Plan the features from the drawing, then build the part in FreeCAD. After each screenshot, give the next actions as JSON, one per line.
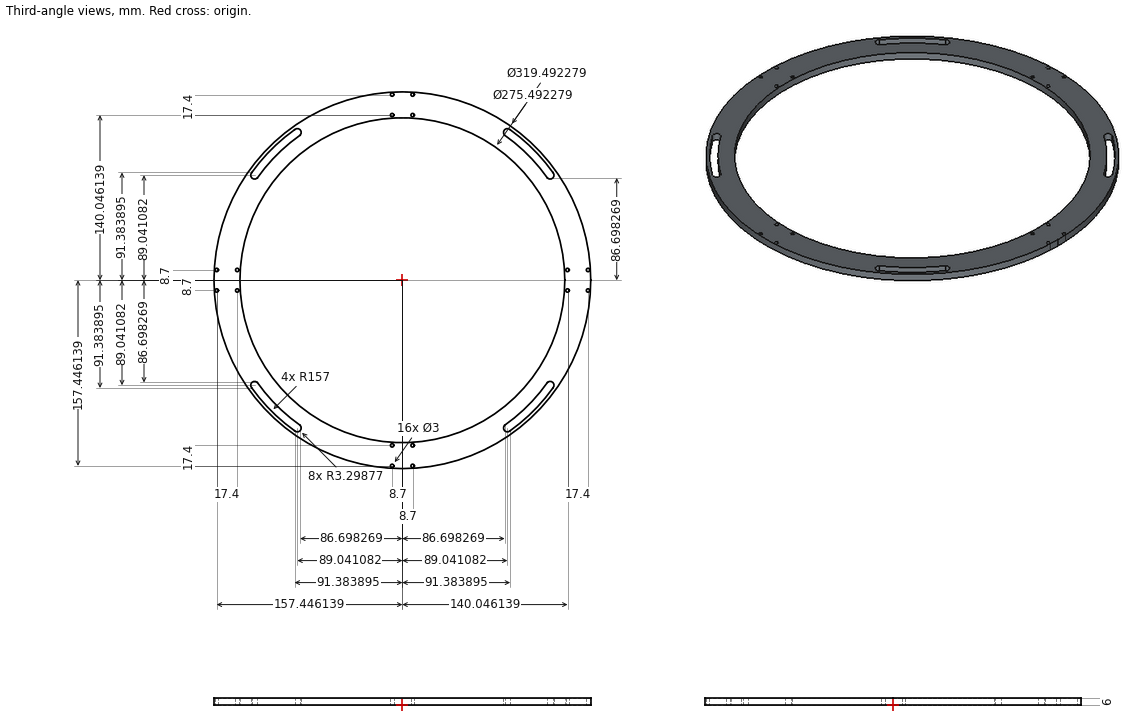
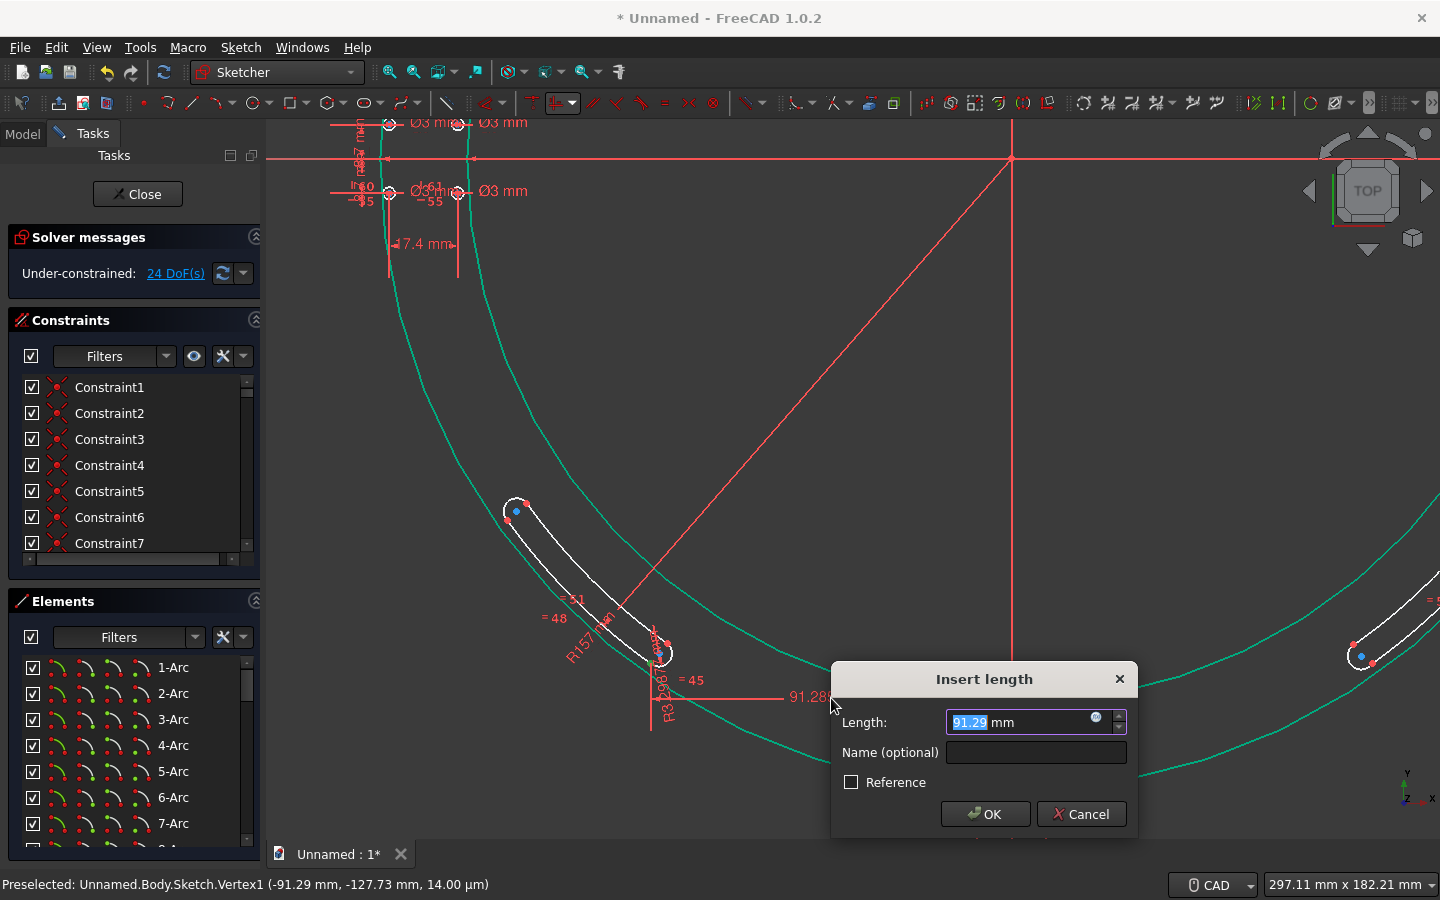
{"action": "type", "text": "91.383895"}
{"action": "key", "text": "Return"}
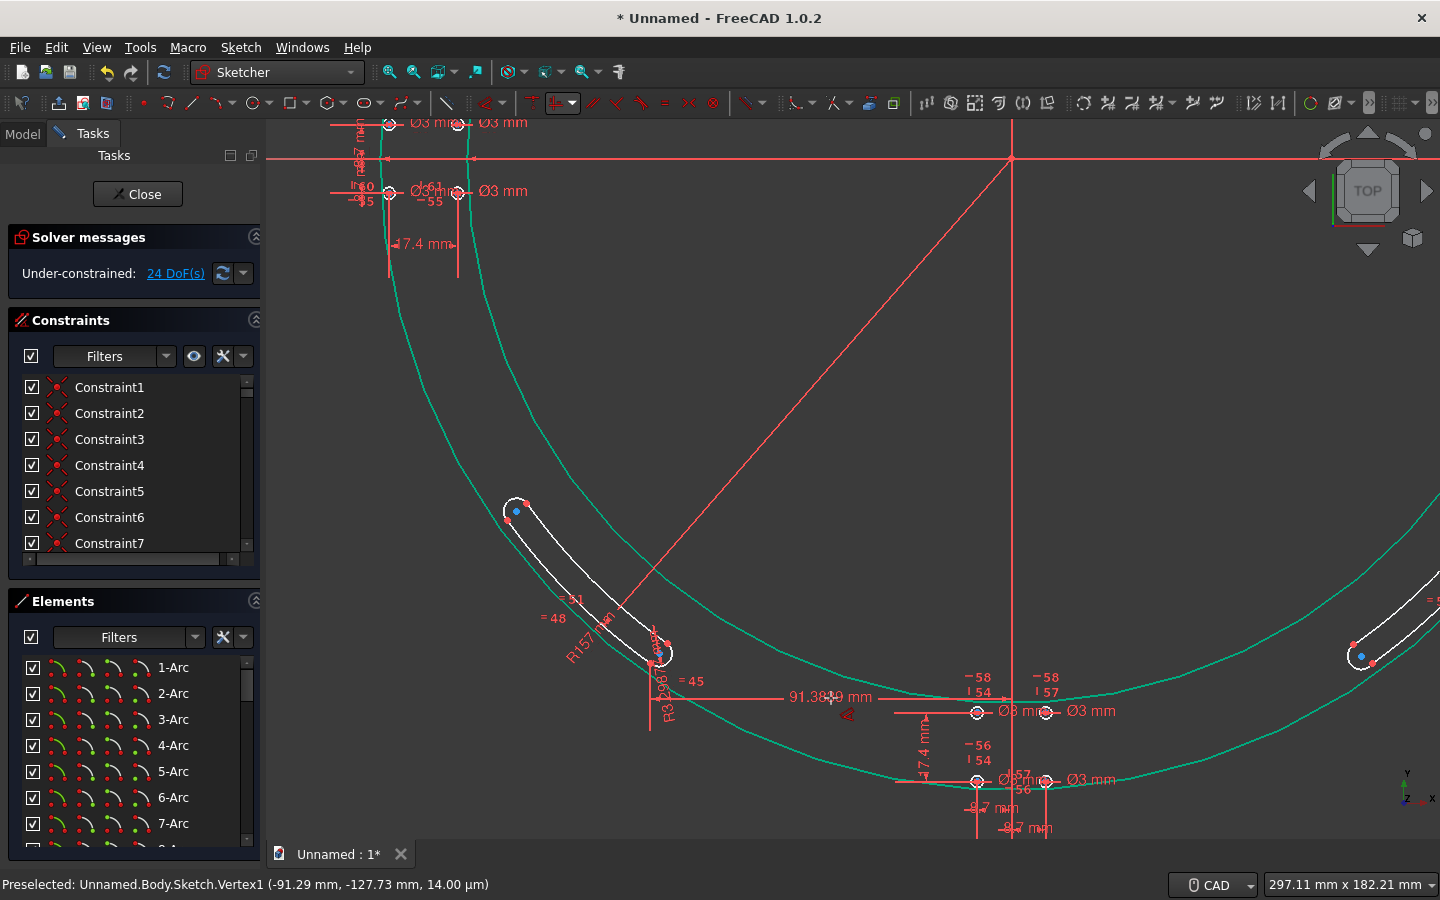
{"action": "left_click", "coordinate": [668, 644]}
{"action": "left_click", "coordinate": [761, 678]}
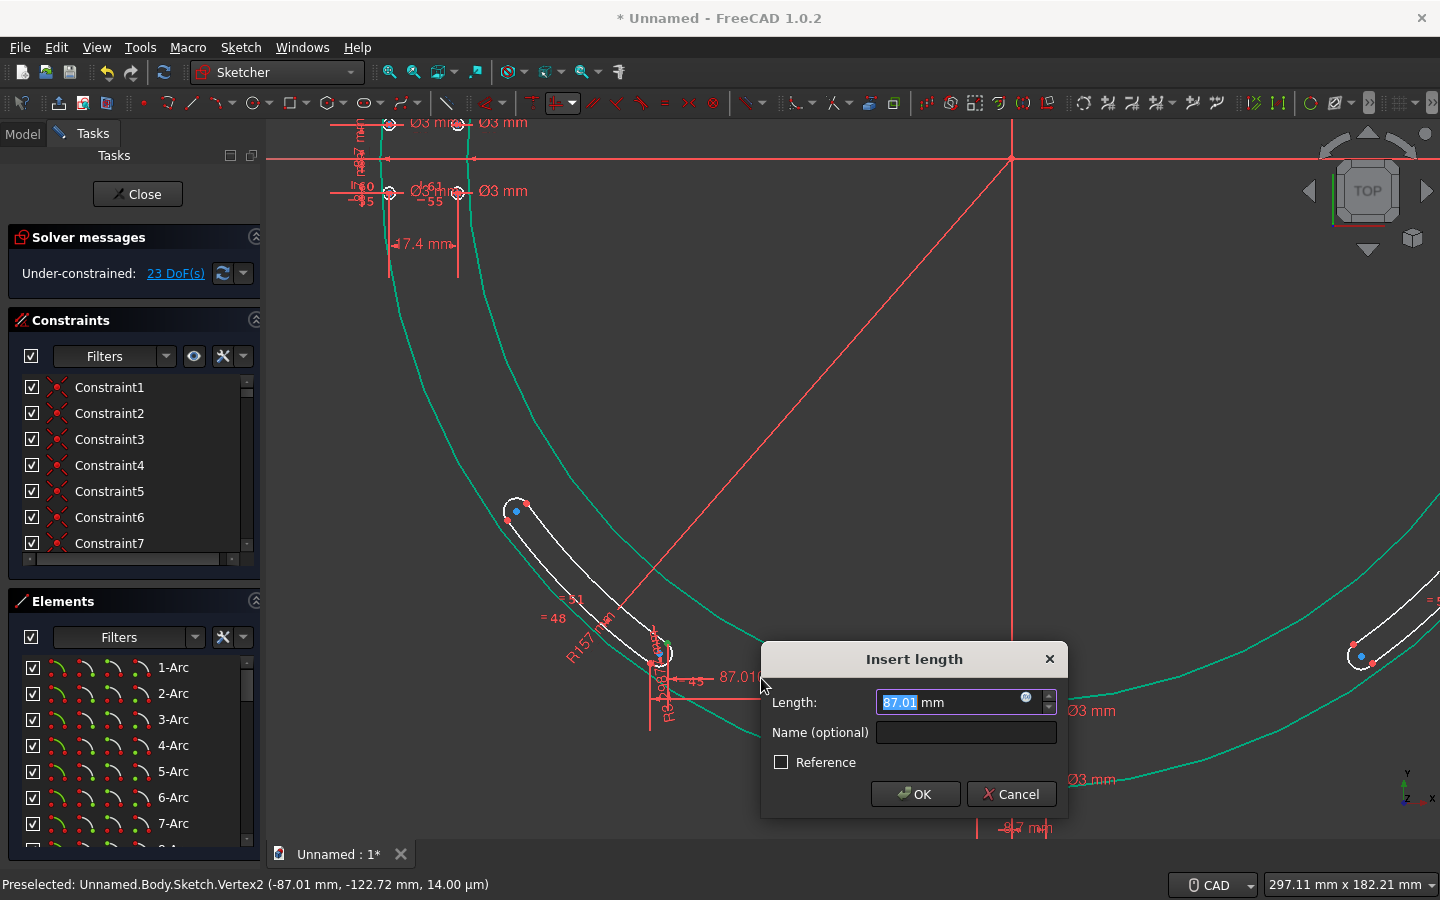
{"action": "type", "text": "86.698269"}
{"action": "key", "text": "Return"}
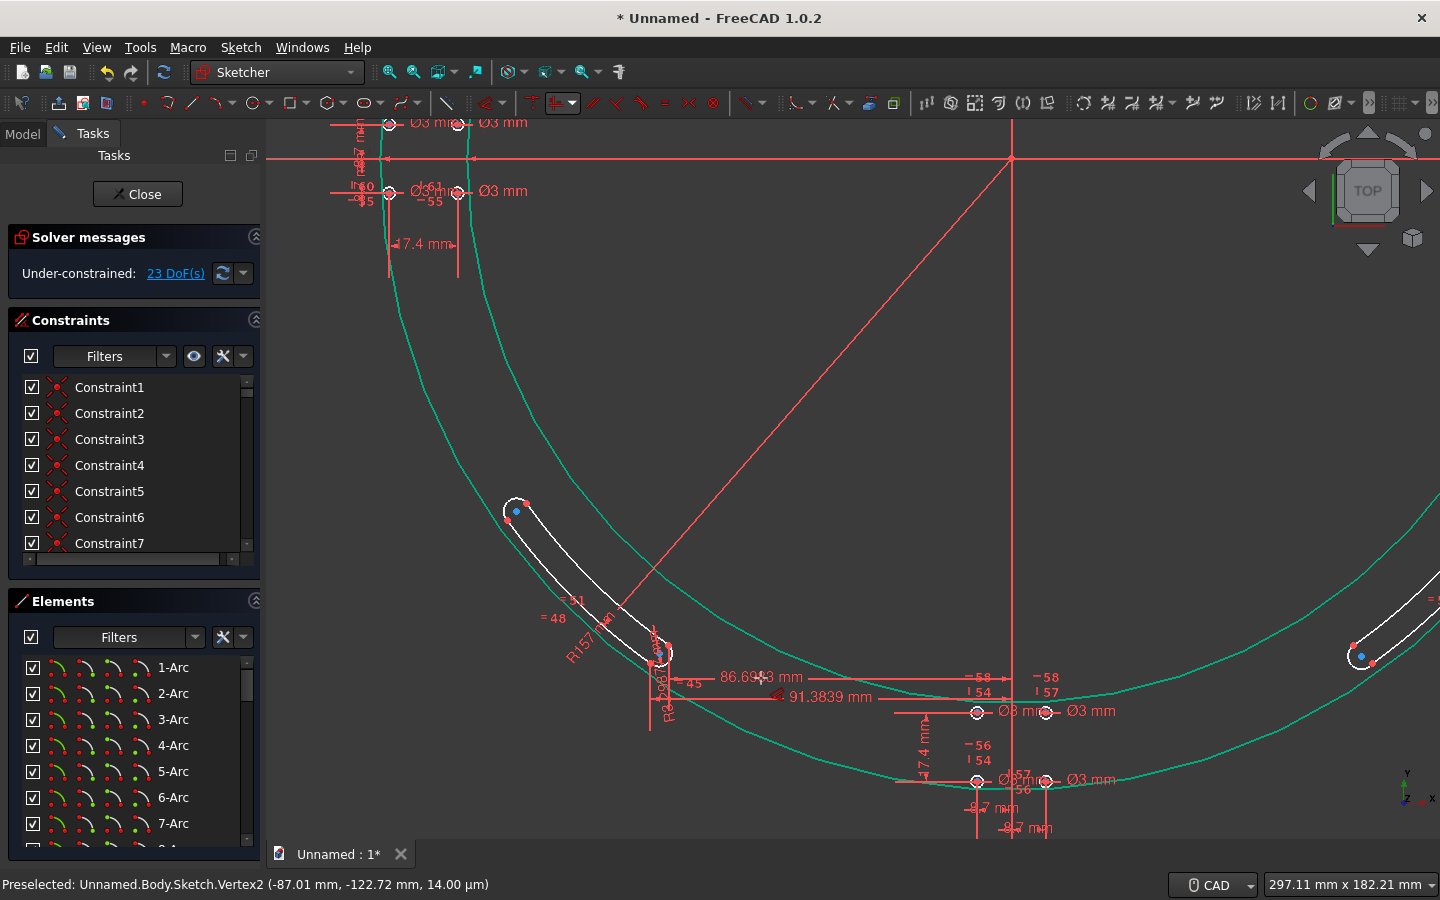
{"action": "left_click", "coordinate": [508, 521]}
{"action": "left_click", "coordinate": [474, 340]}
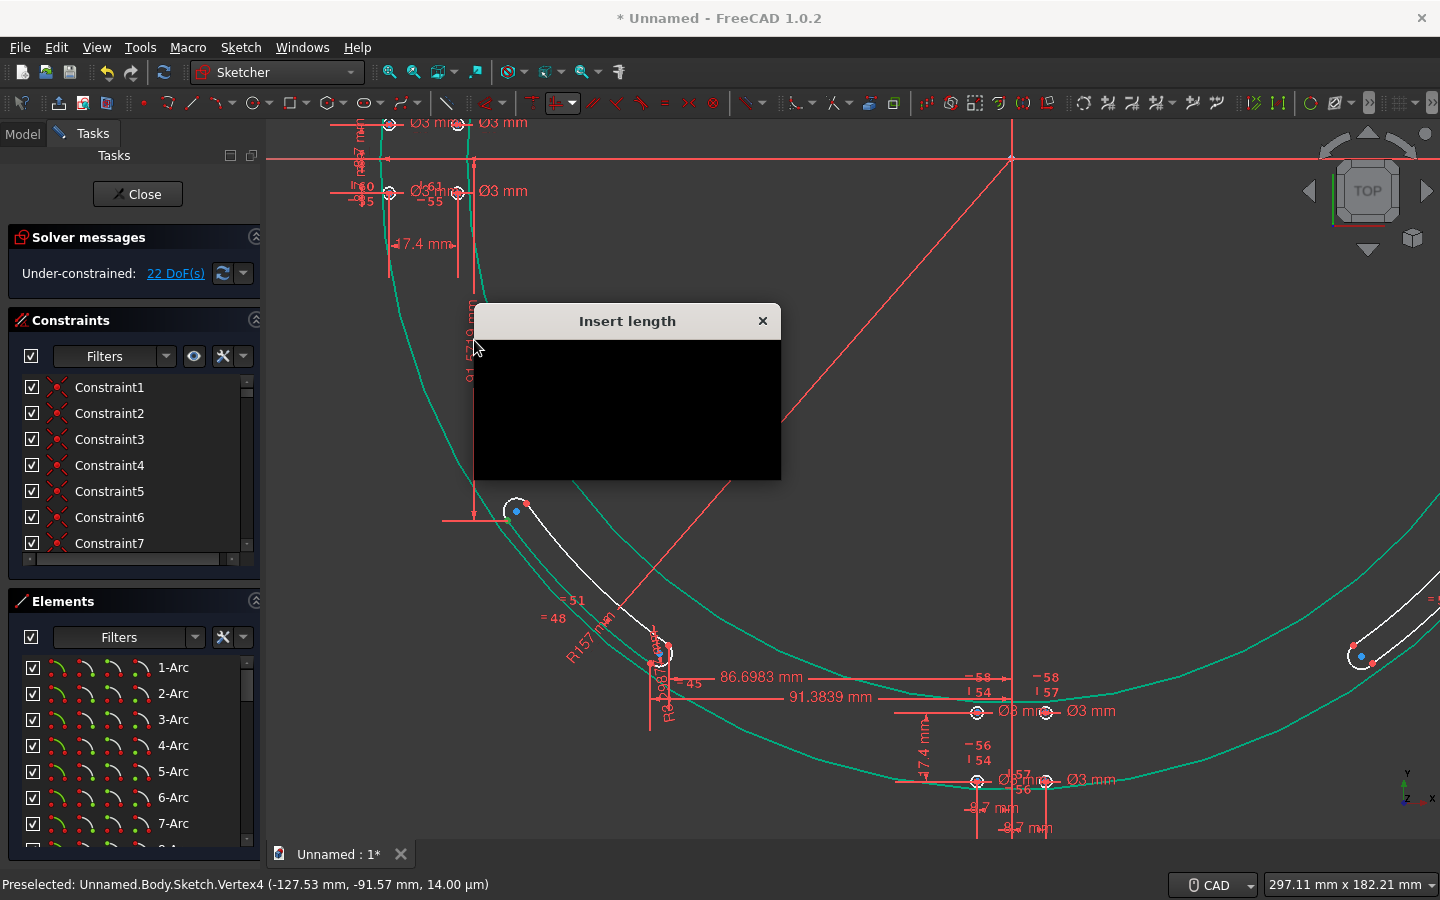
{"action": "type", "text": "91.383895"}
{"action": "key", "text": "Return"}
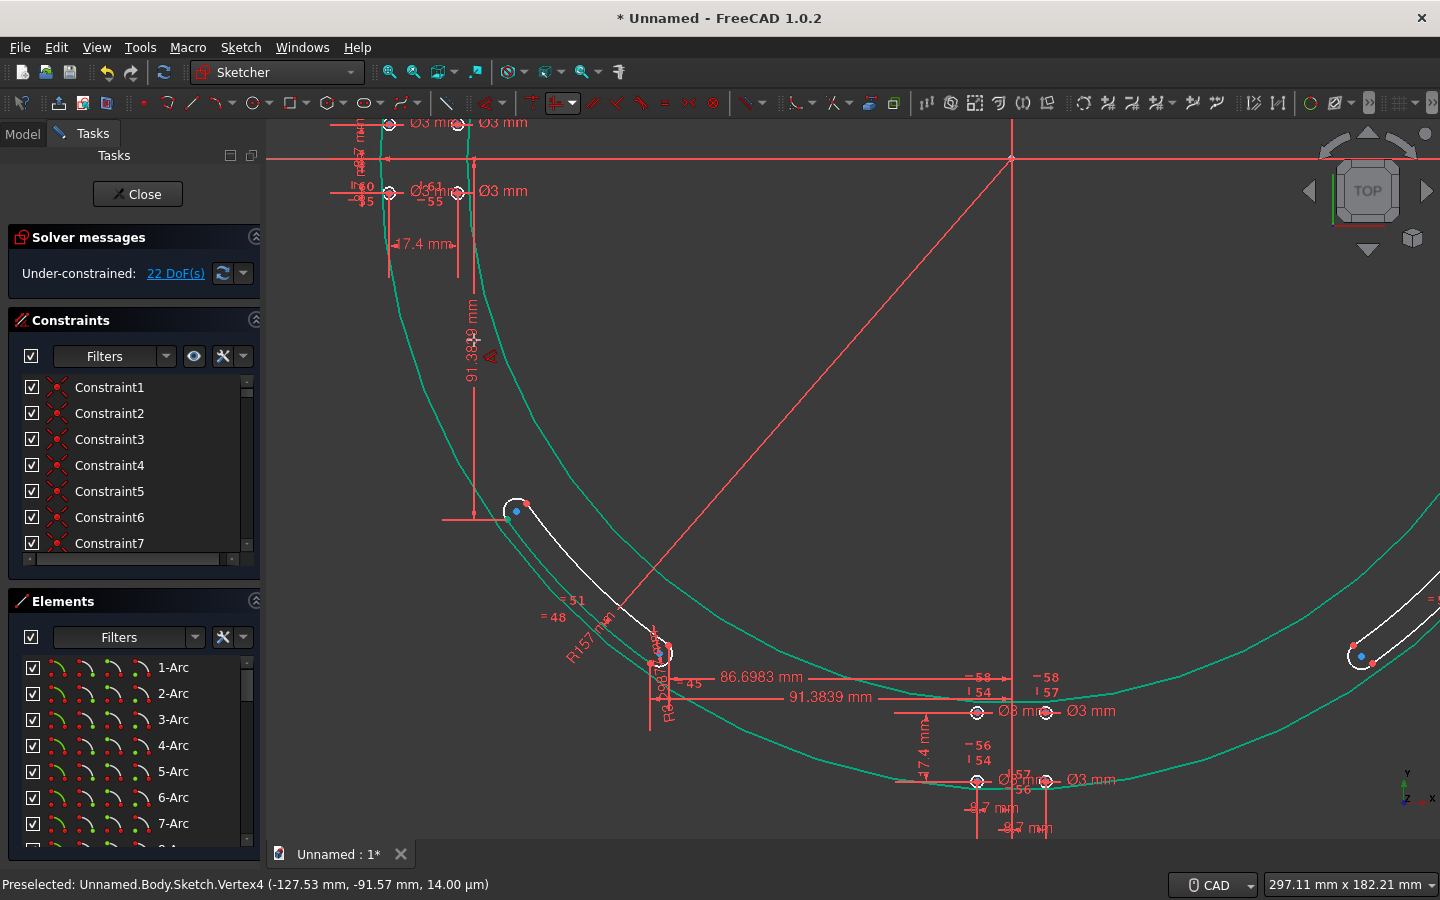
{"action": "left_click", "coordinate": [526, 503]}
{"action": "left_click", "coordinate": [492, 410]}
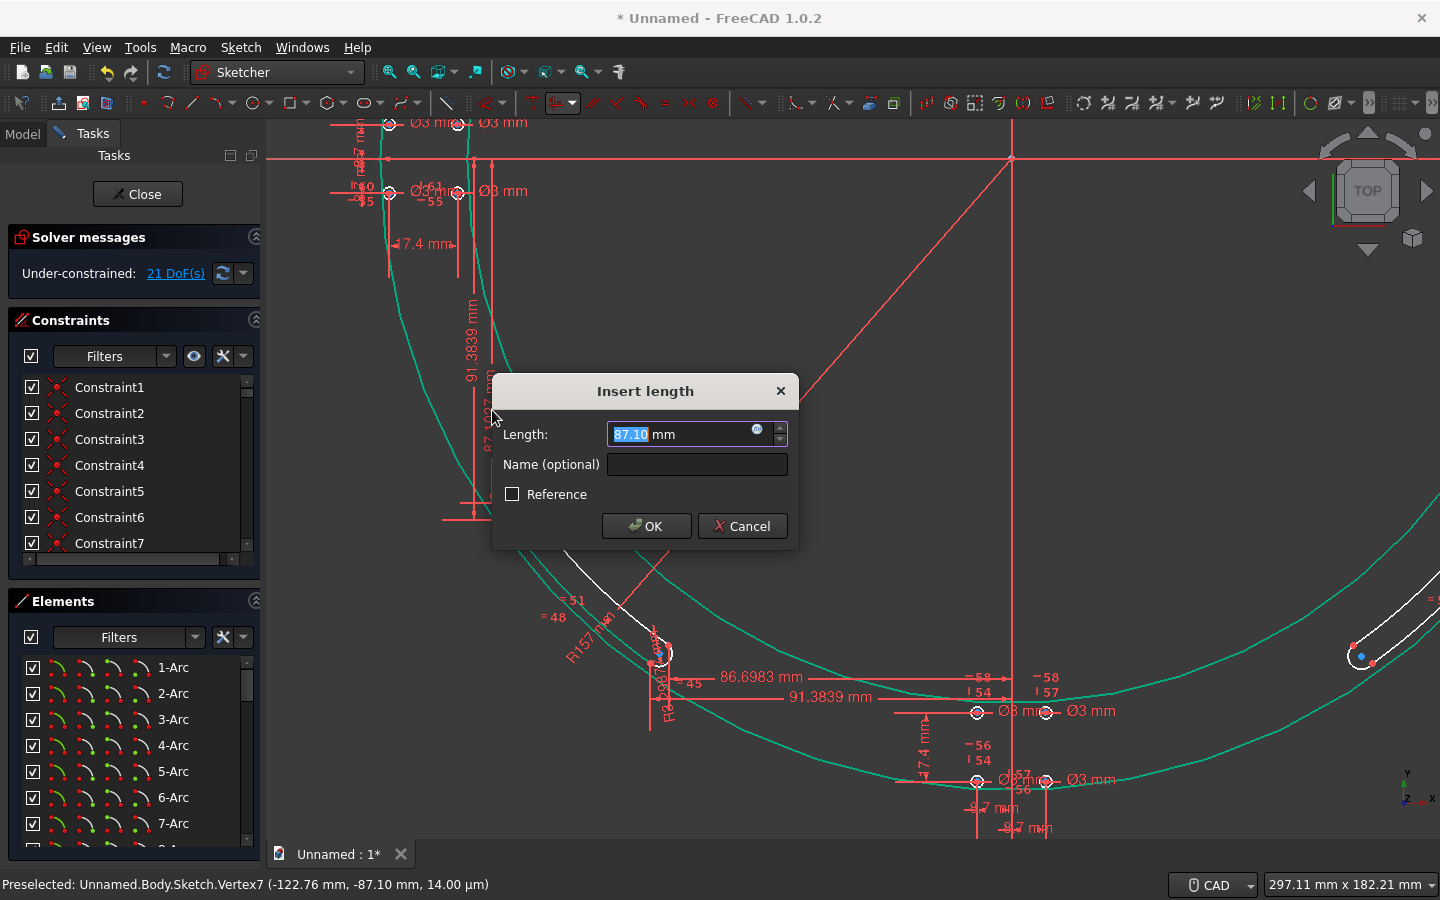
{"action": "type", "text": "86.698269"}
{"action": "key", "text": "Return"}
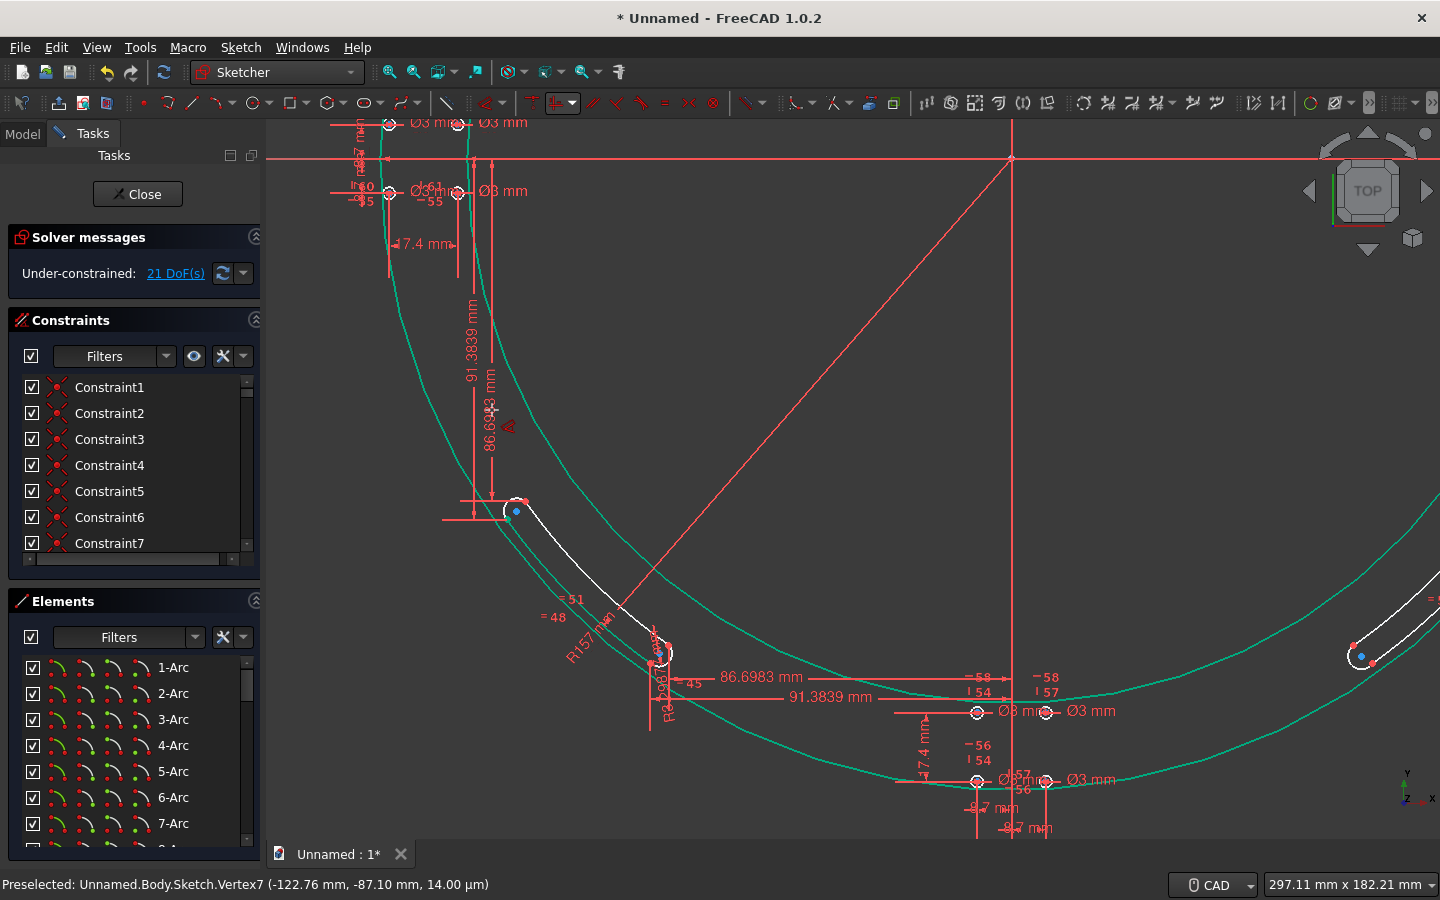
{"action": "scroll", "coordinate": [652, 665], "scroll_direction": "down", "scroll_amount": 5}